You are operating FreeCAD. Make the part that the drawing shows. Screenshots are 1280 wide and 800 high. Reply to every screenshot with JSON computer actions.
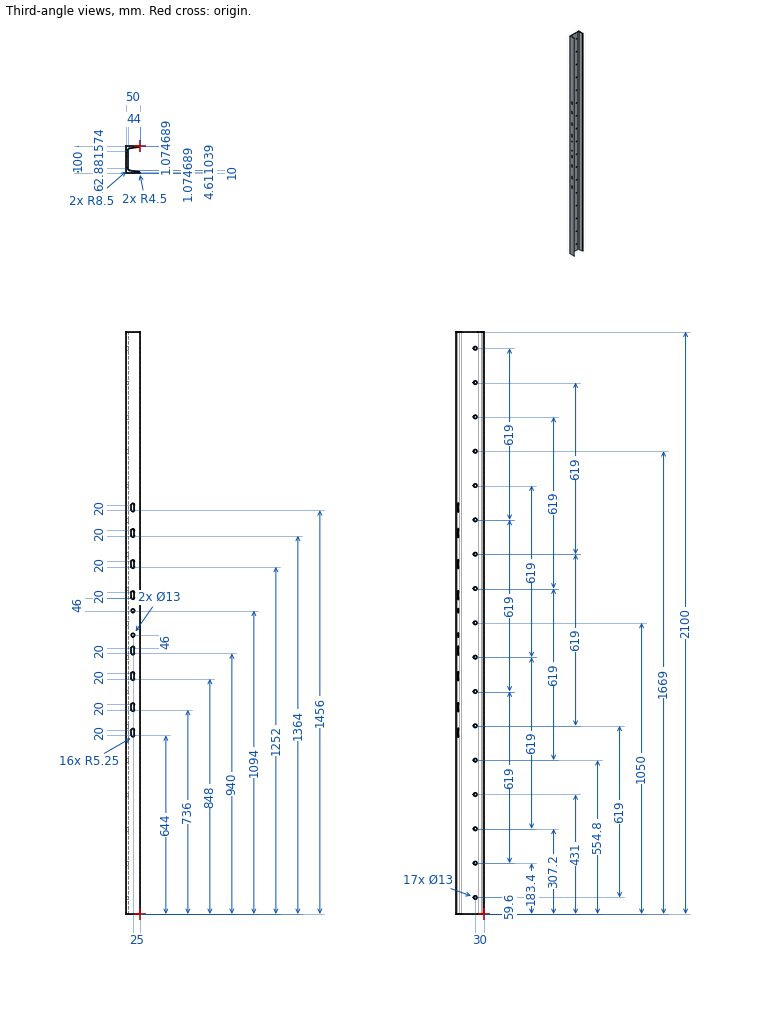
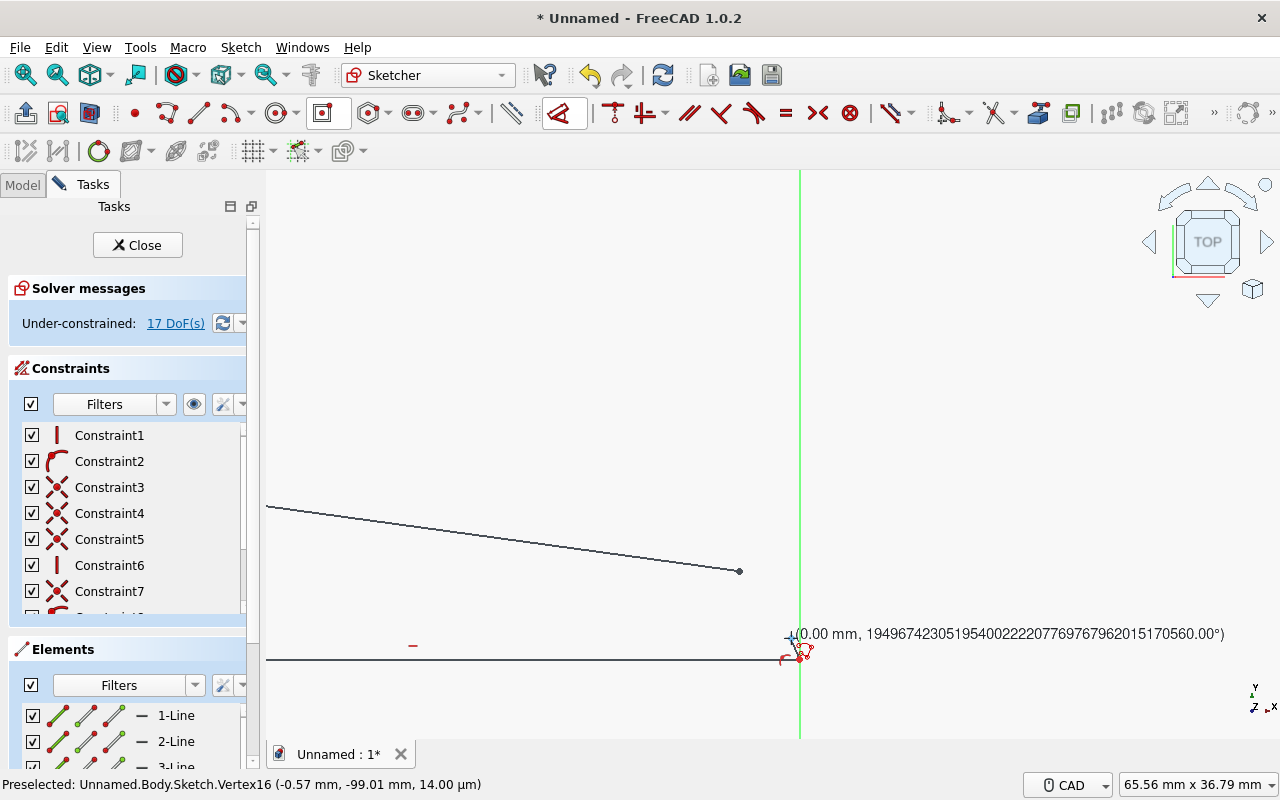
{"action": "left_click", "coordinate": [254, 114]}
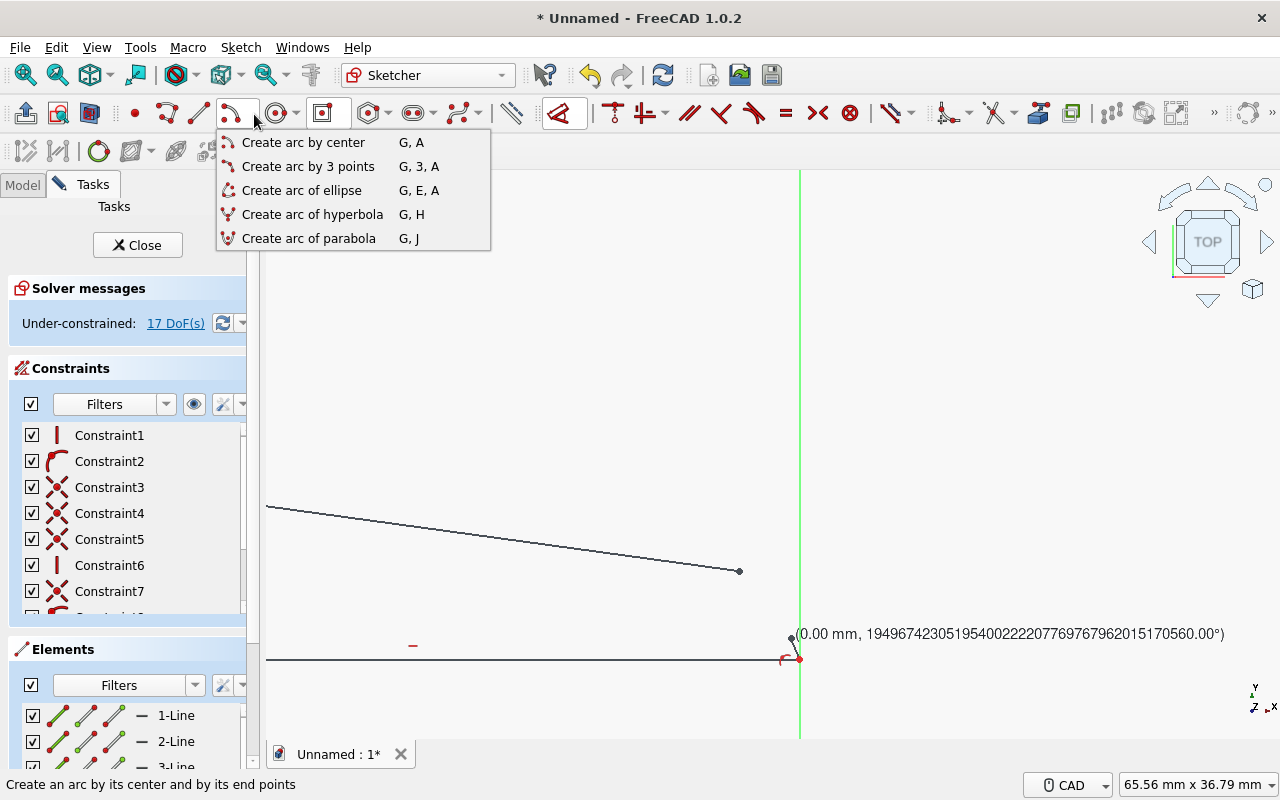
{"action": "left_click", "coordinate": [354, 166]}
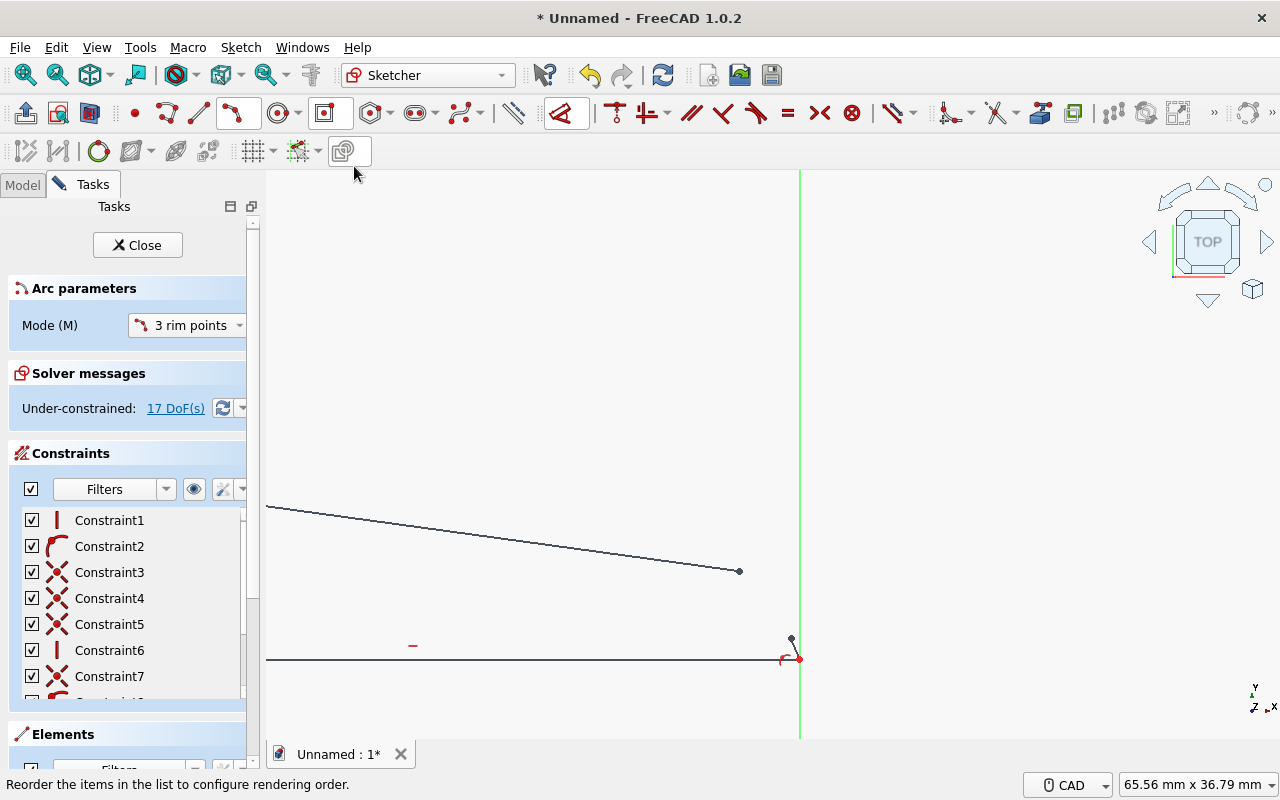
{"action": "scroll", "coordinate": [800, 642], "scroll_direction": "down", "scroll_amount": 7}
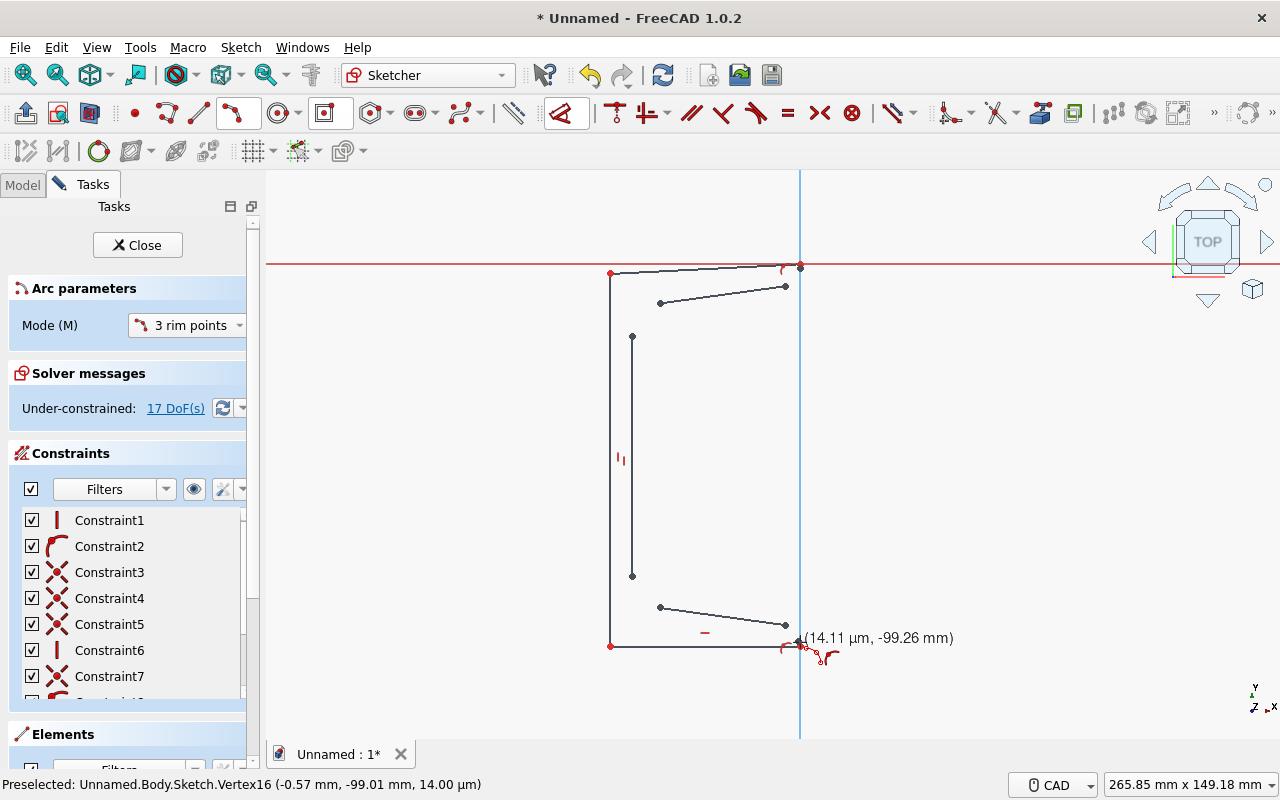
{"action": "left_click", "coordinate": [660, 608]}
{"action": "left_click", "coordinate": [632, 576]}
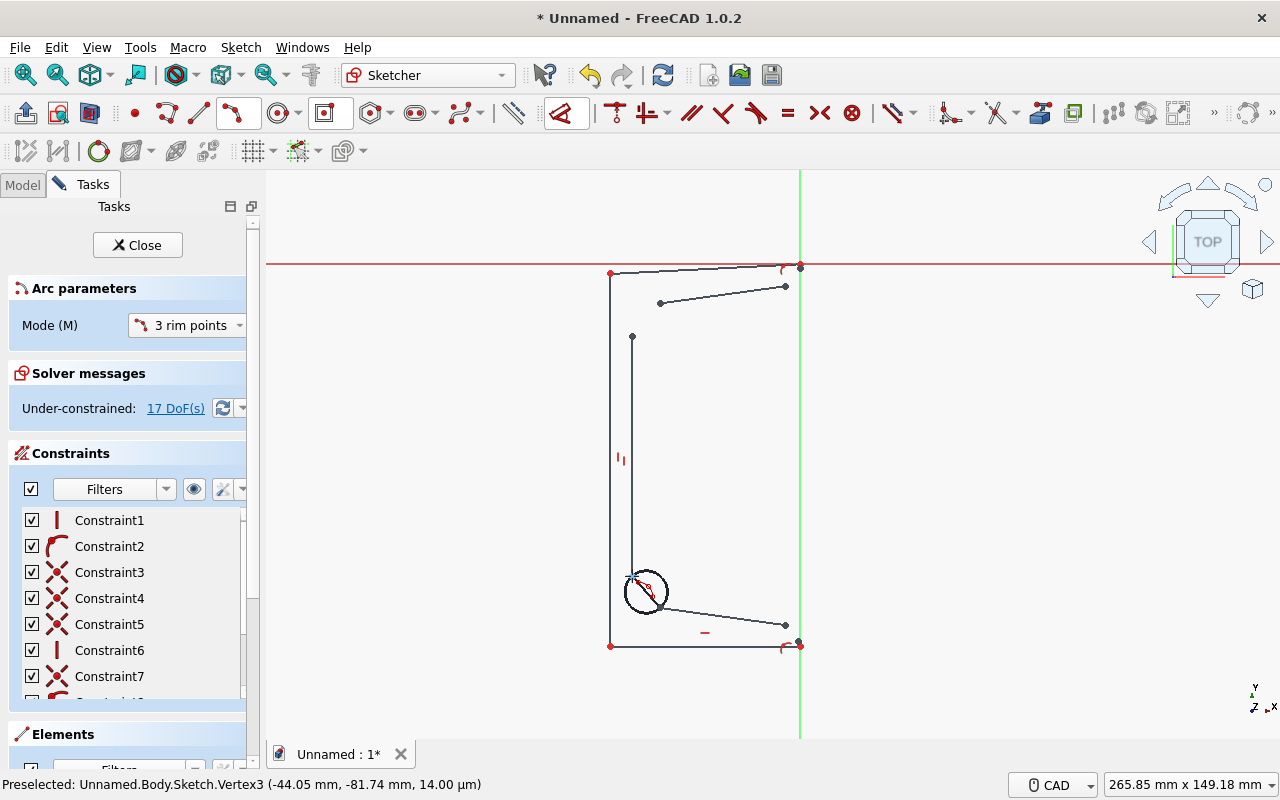
{"action": "scroll", "coordinate": [640, 596], "scroll_direction": "up", "scroll_amount": 4}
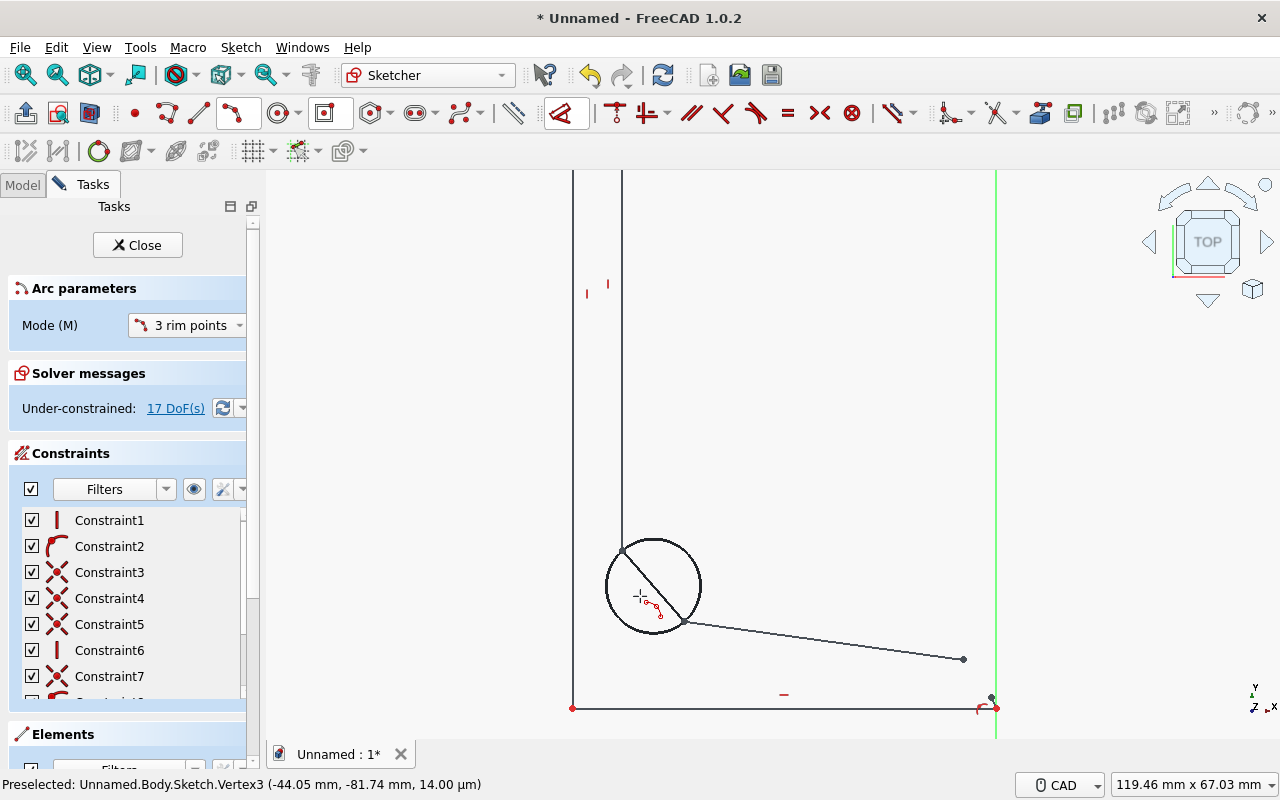
{"action": "left_click", "coordinate": [641, 595]}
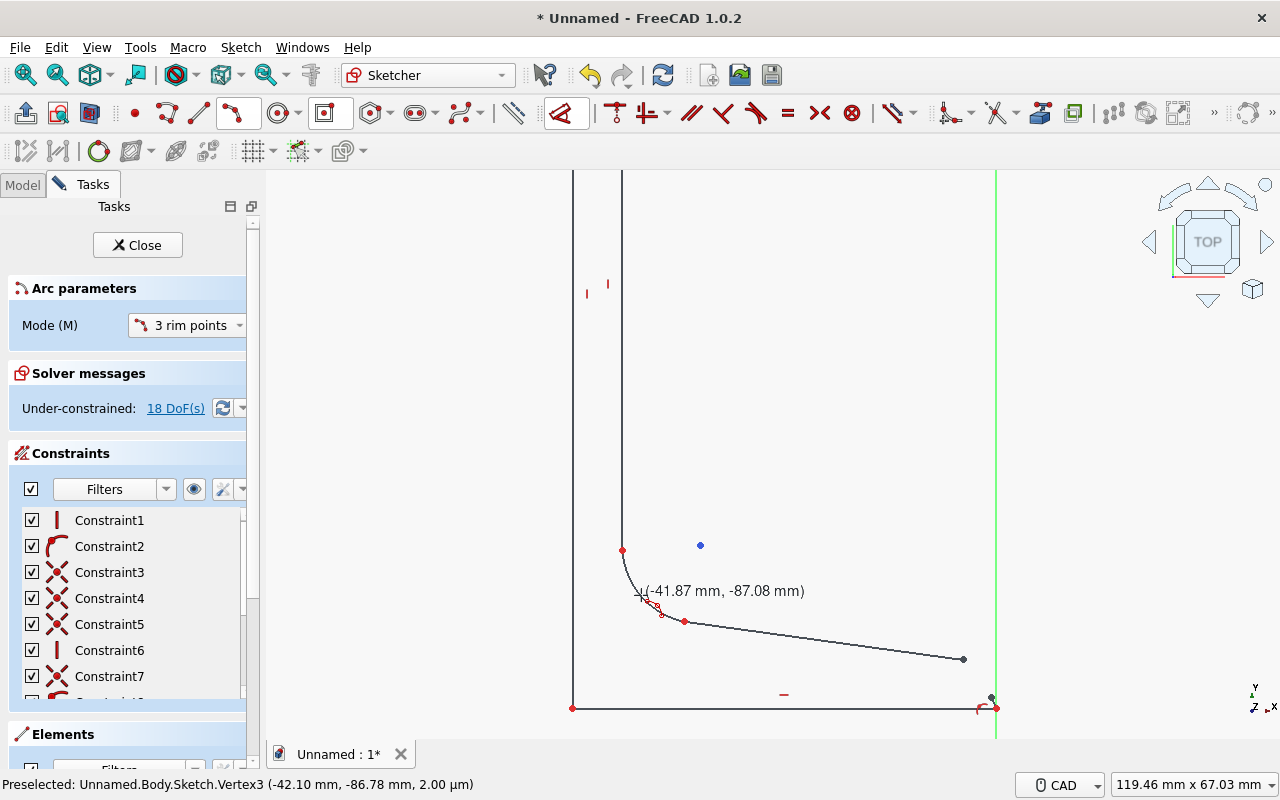
{"action": "scroll", "coordinate": [639, 596], "scroll_direction": "down", "scroll_amount": 4}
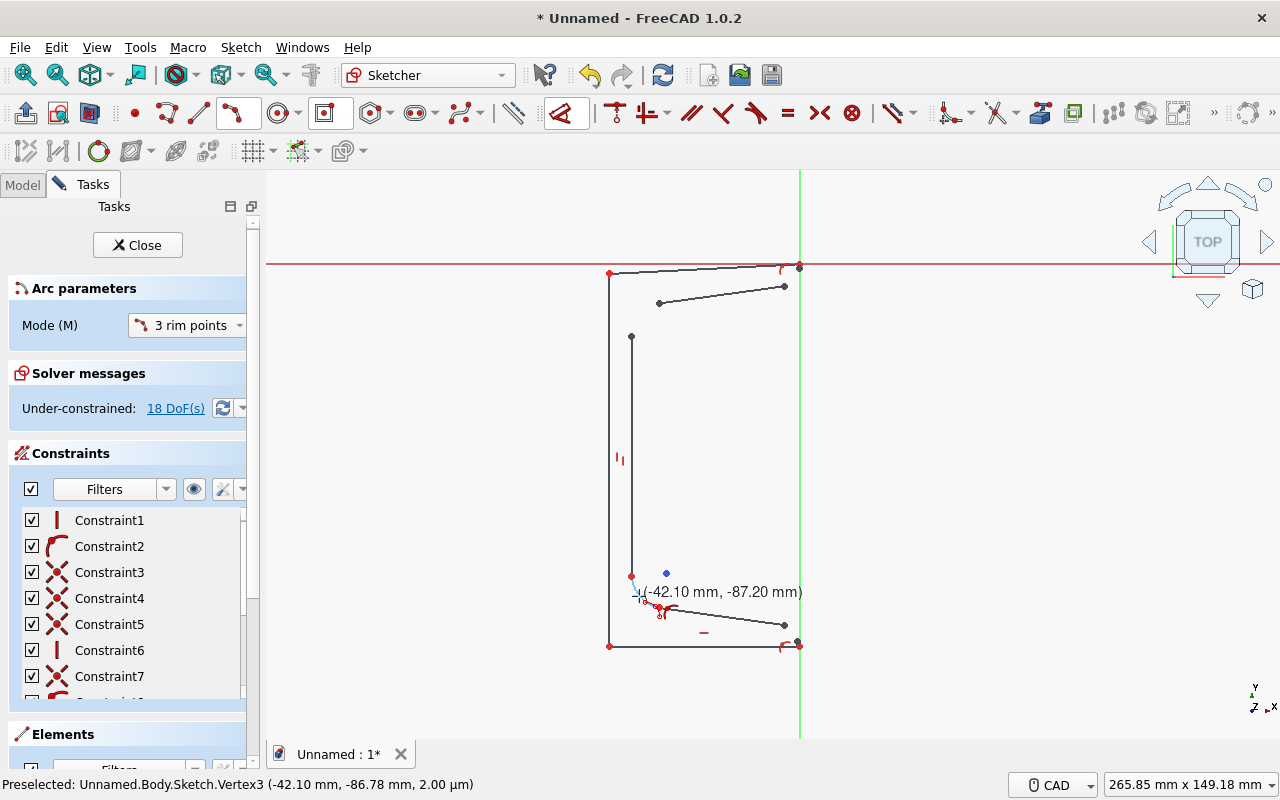
{"action": "left_click", "coordinate": [632, 336]}
{"action": "left_click", "coordinate": [660, 303]}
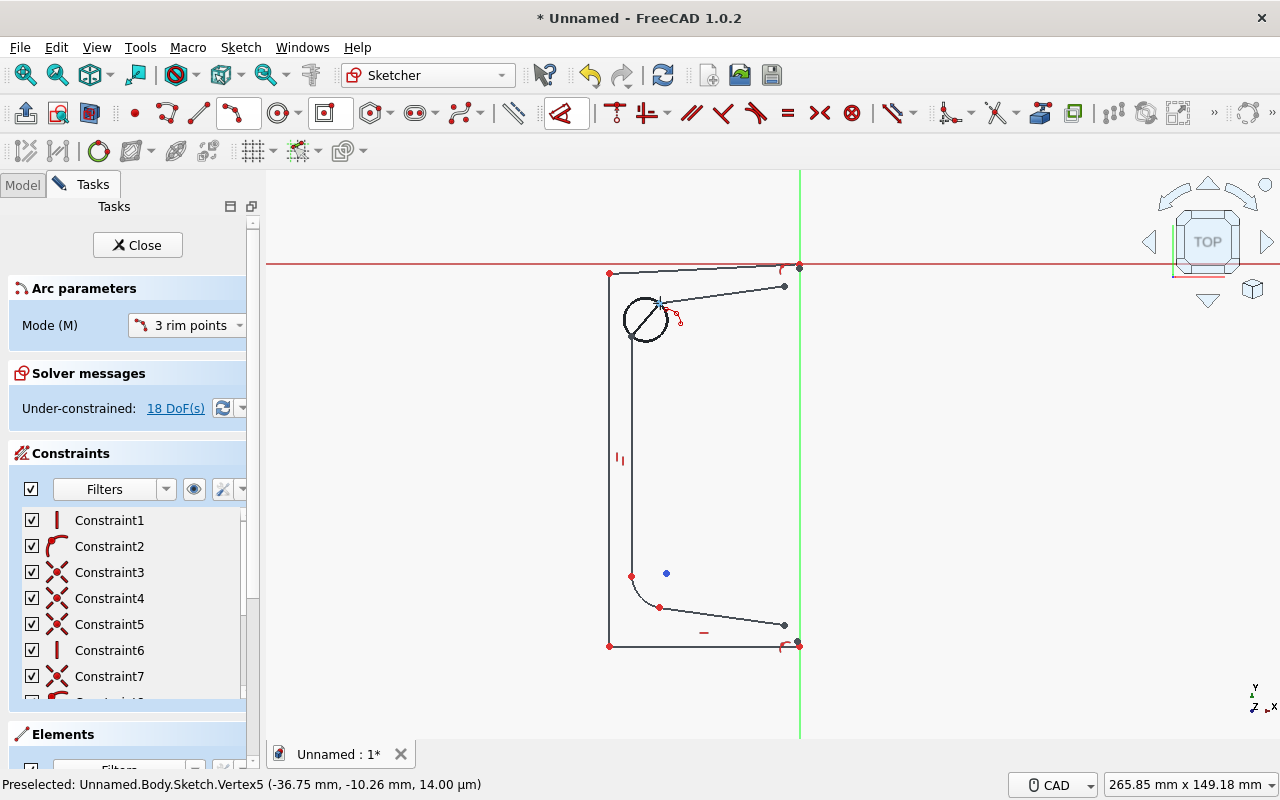
{"action": "scroll", "coordinate": [640, 314], "scroll_direction": "up", "scroll_amount": 4}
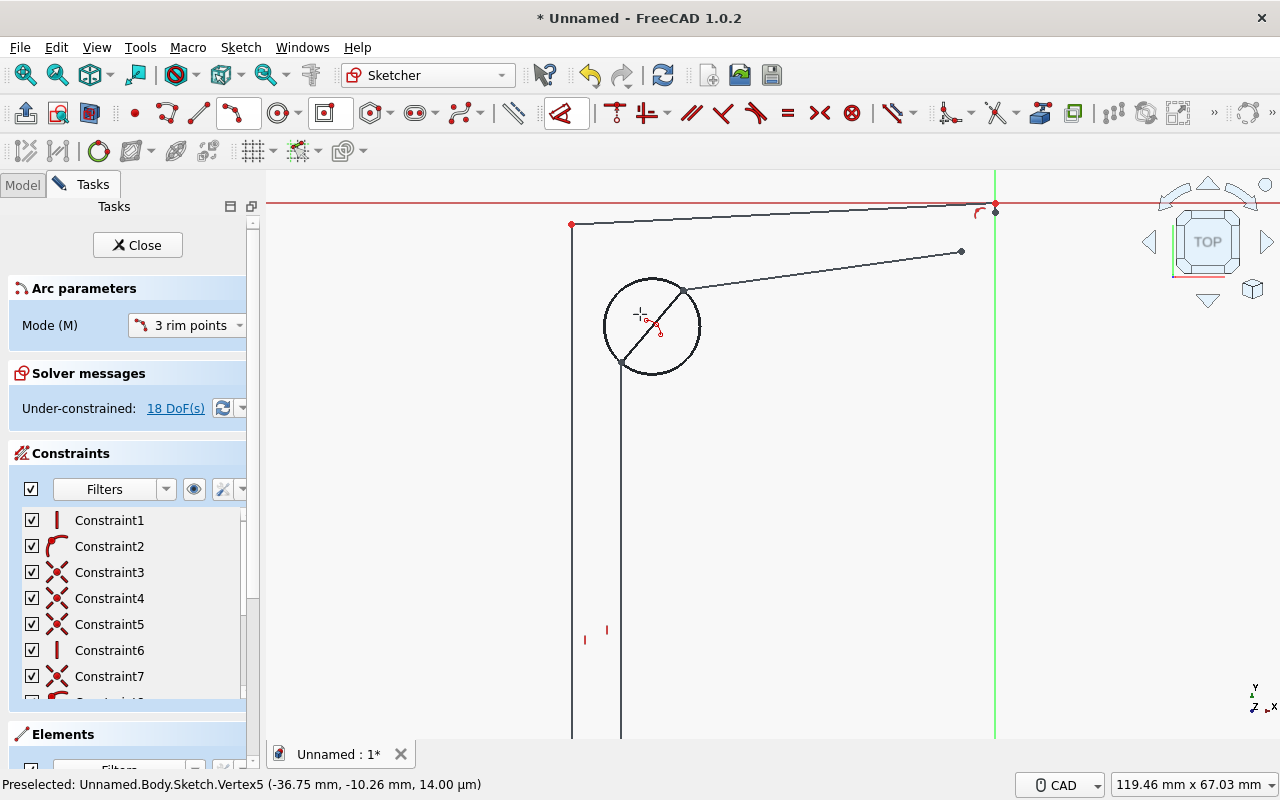
{"action": "left_click", "coordinate": [639, 313]}